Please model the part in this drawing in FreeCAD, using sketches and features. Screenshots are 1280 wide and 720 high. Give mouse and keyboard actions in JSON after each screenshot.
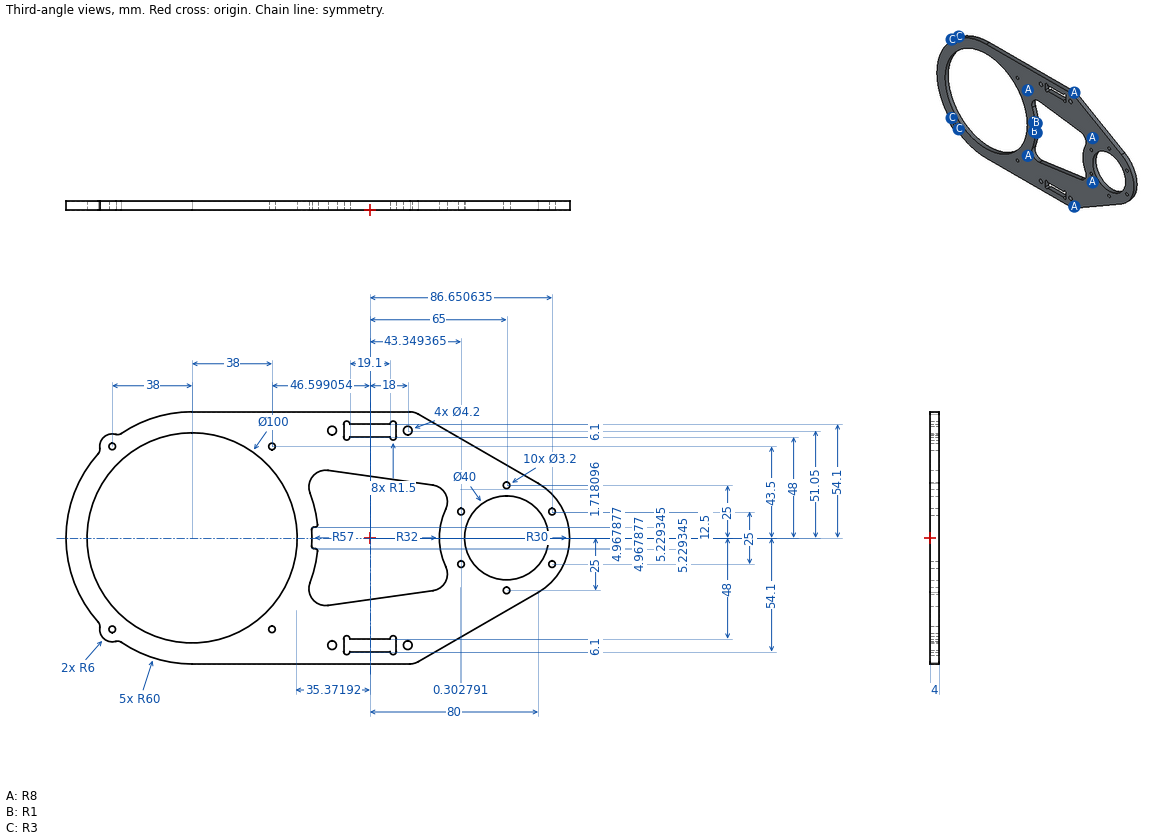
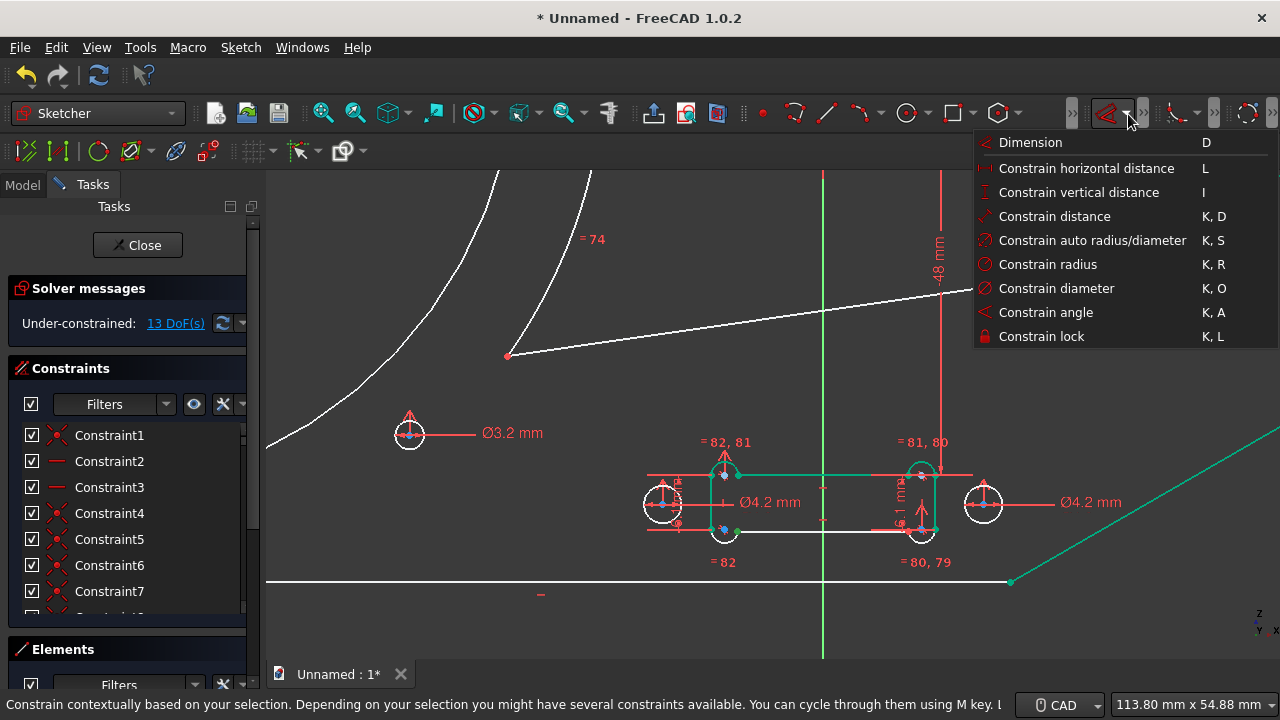
{"action": "left_click", "coordinate": [1126, 192]}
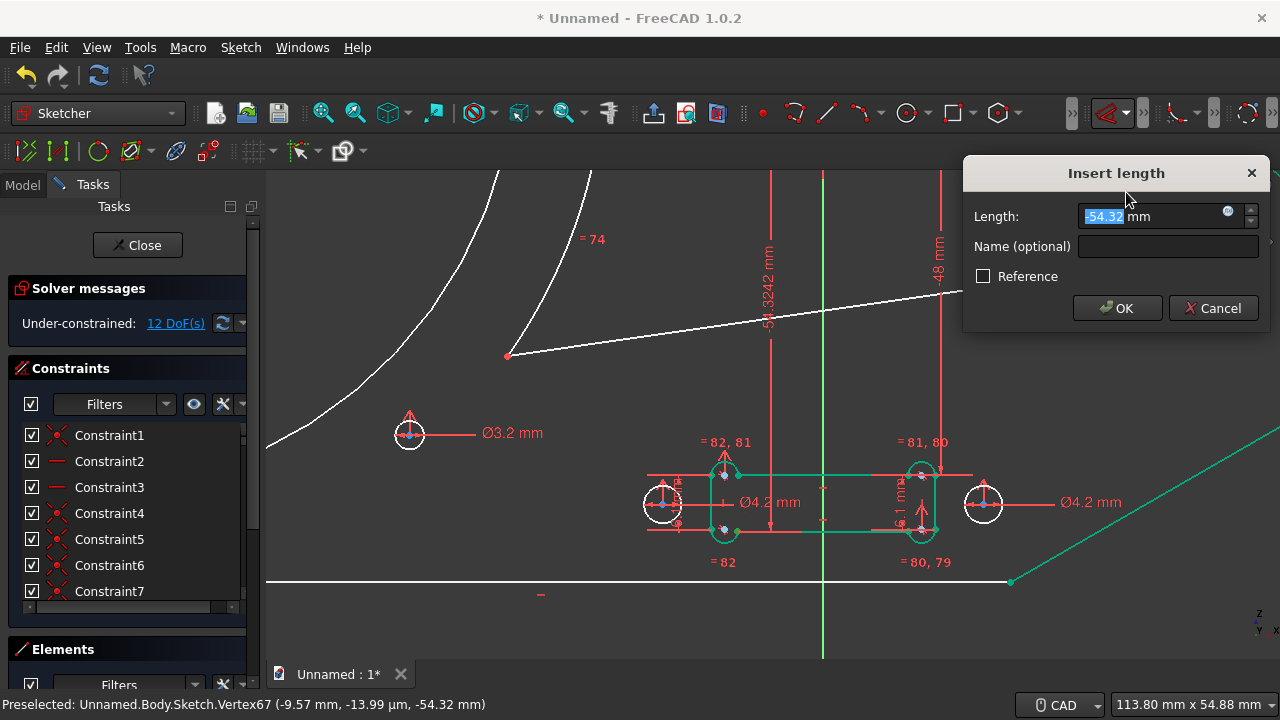
{"action": "type", "text": "-54.1"}
{"action": "key", "text": "Return"}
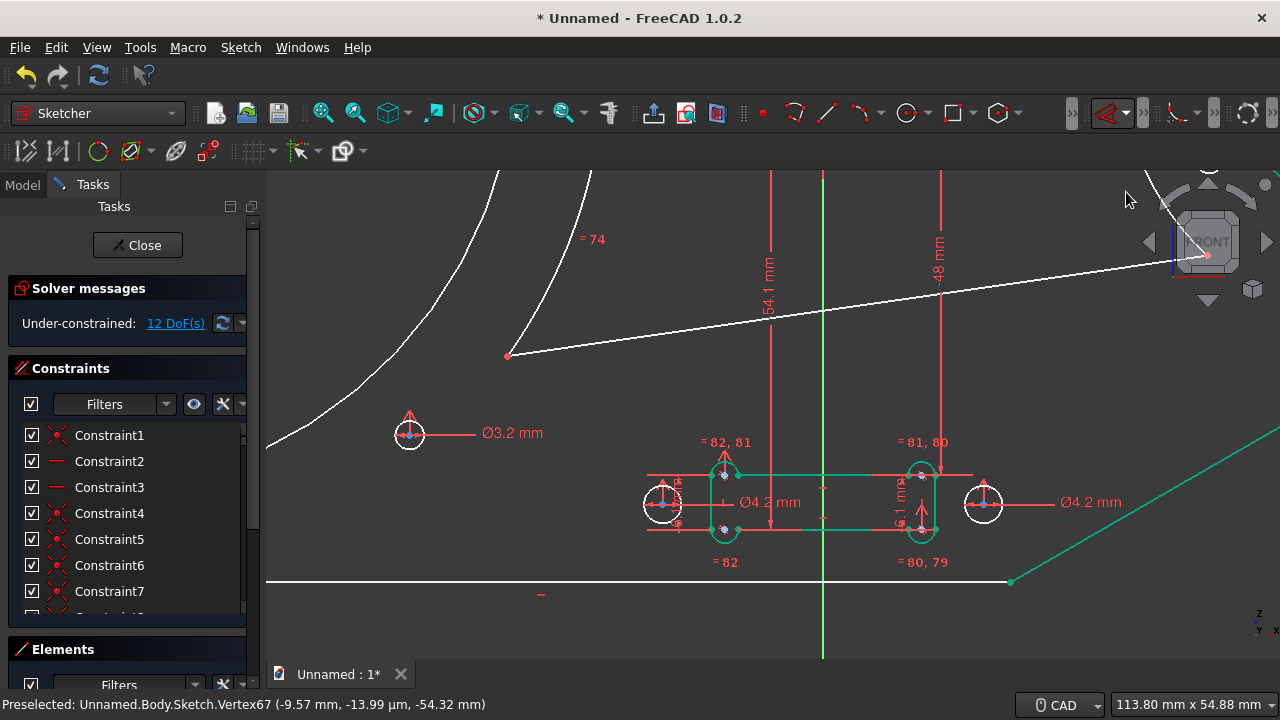
{"action": "scroll", "coordinate": [738, 535], "scroll_direction": "down", "scroll_amount": 7}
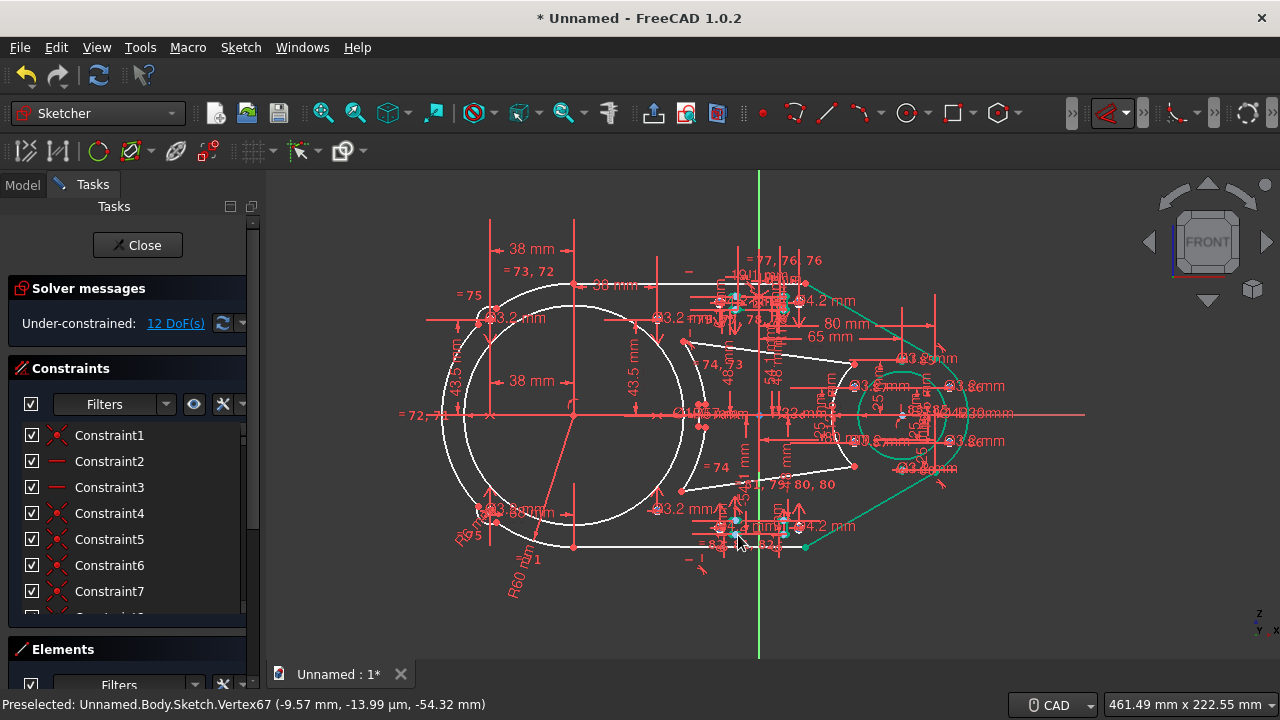
{"action": "left_click", "coordinate": [799, 303]}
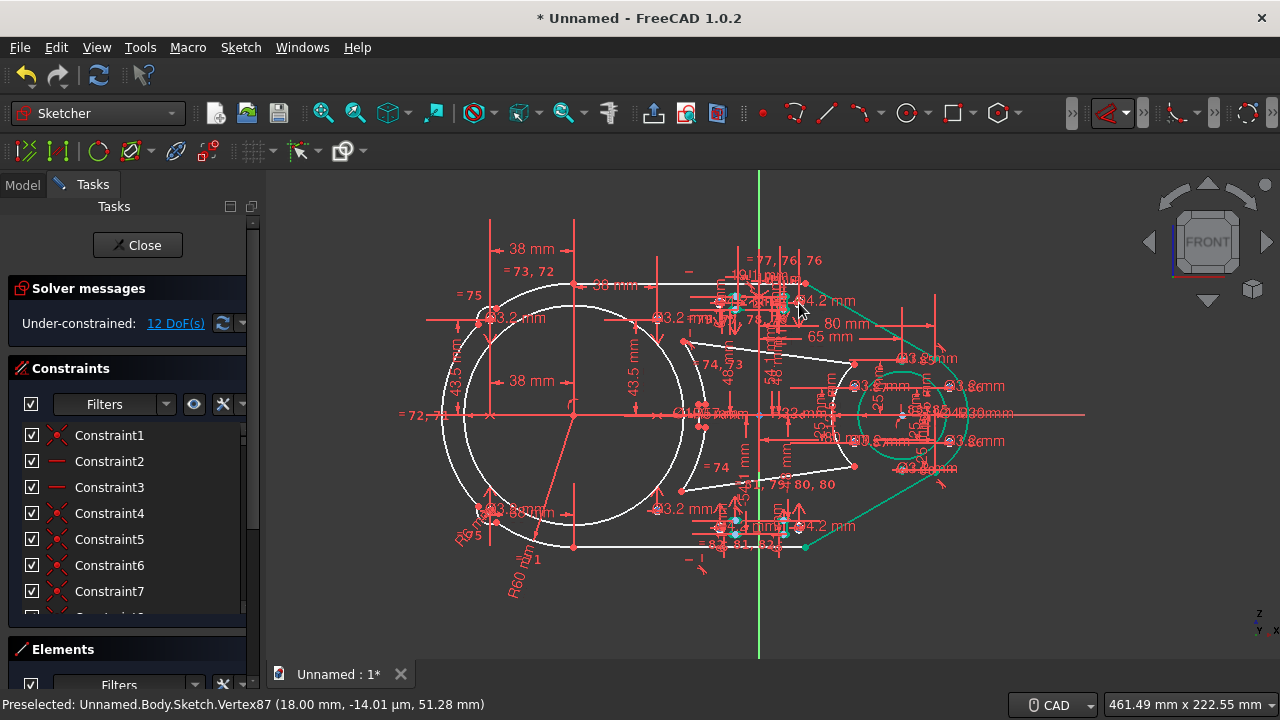
{"action": "key", "text": "i"}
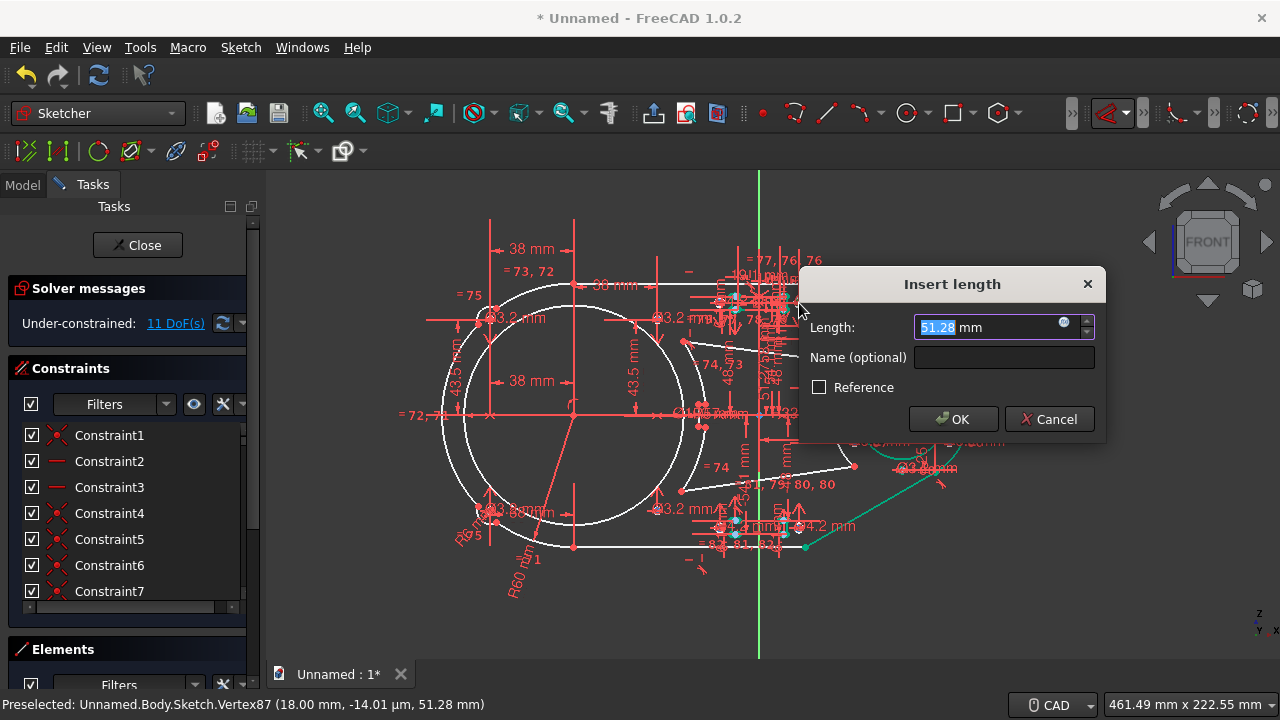
{"action": "type", "text": "51.05"}
{"action": "key", "text": "Return"}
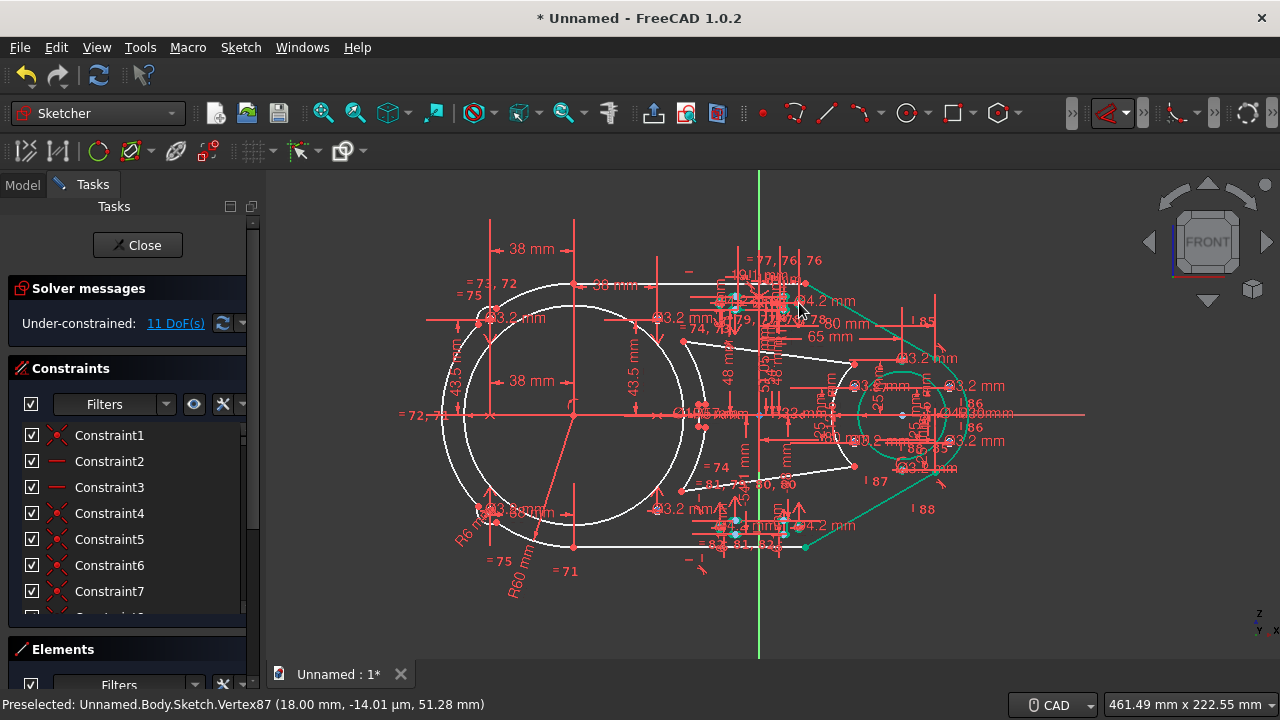
{"action": "left_click", "coordinate": [682, 491]}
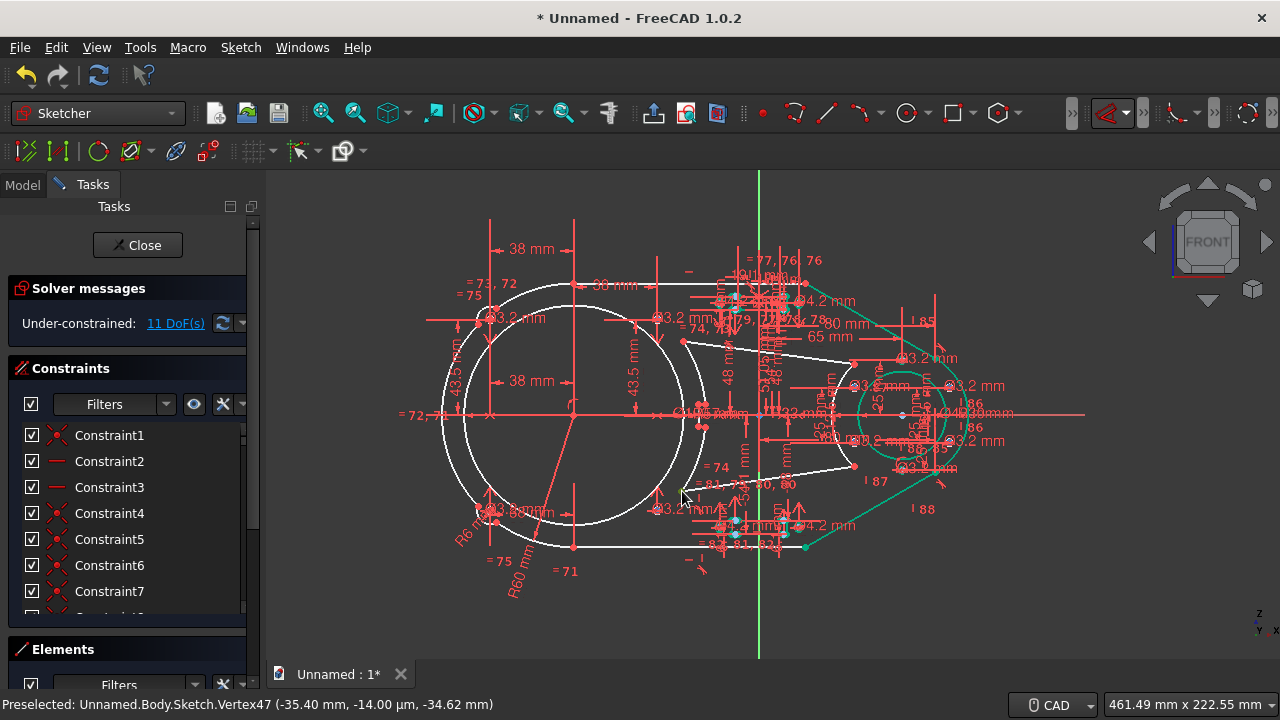
{"action": "left_click", "coordinate": [1128, 114]}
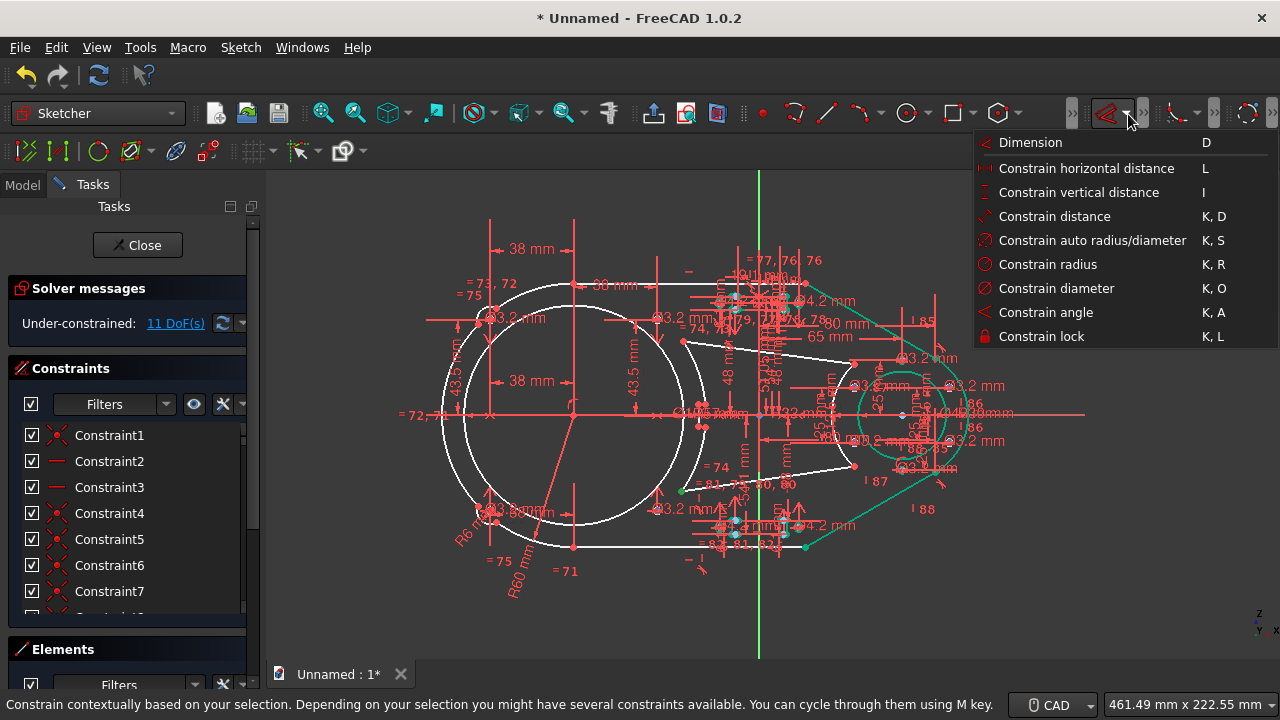
{"action": "left_click", "coordinate": [1126, 168]}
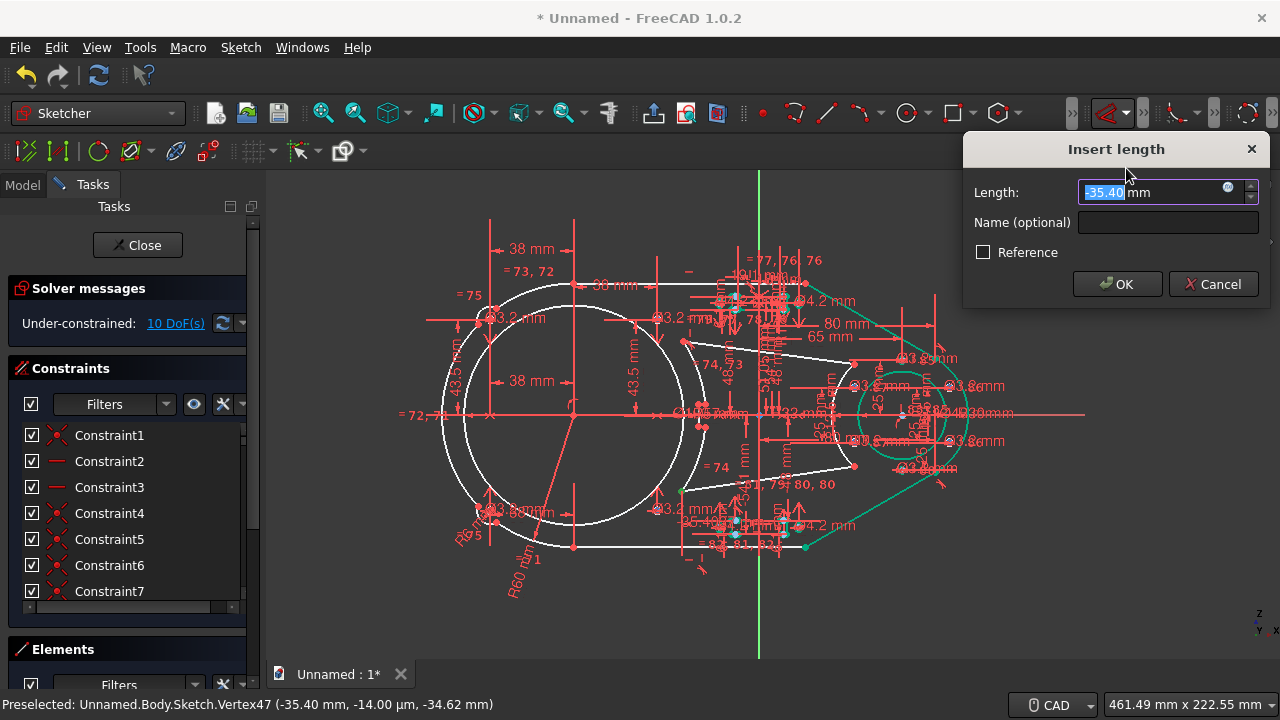
{"action": "type", "text": "-35.37192"}
{"action": "key", "text": "Return"}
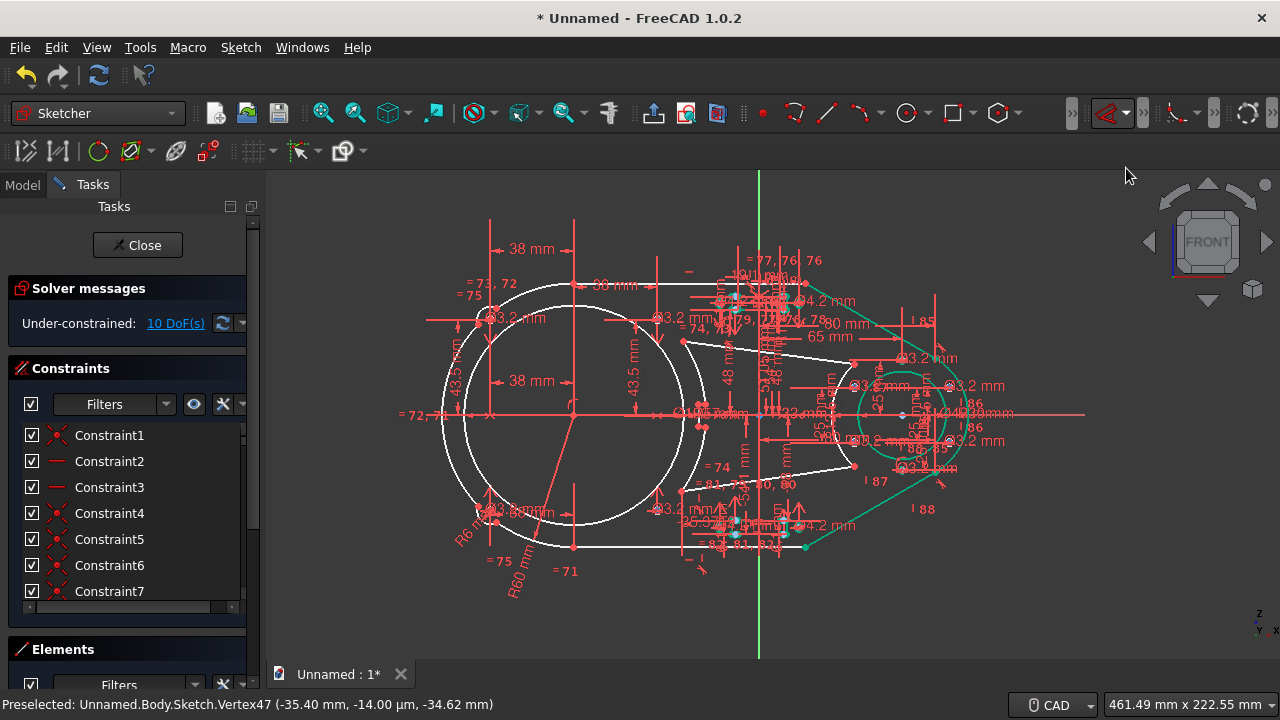
{"action": "left_click", "coordinate": [683, 342]}